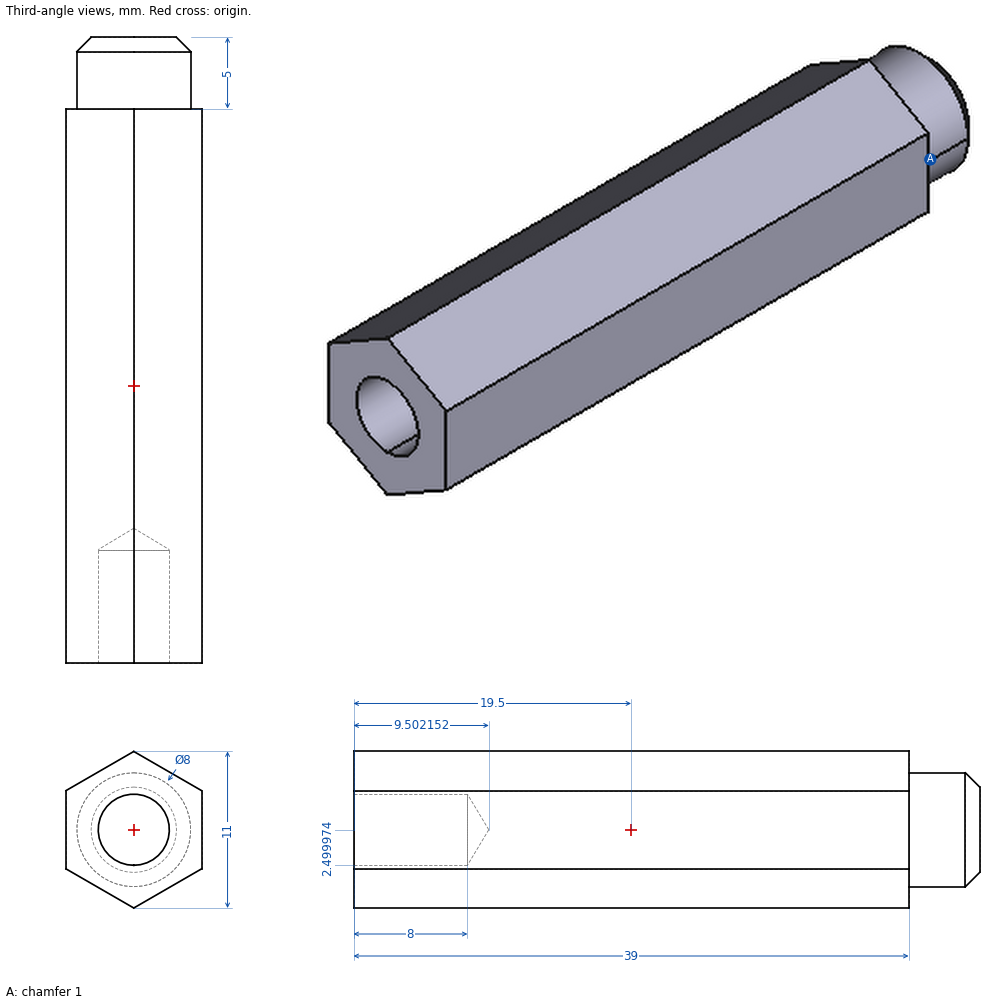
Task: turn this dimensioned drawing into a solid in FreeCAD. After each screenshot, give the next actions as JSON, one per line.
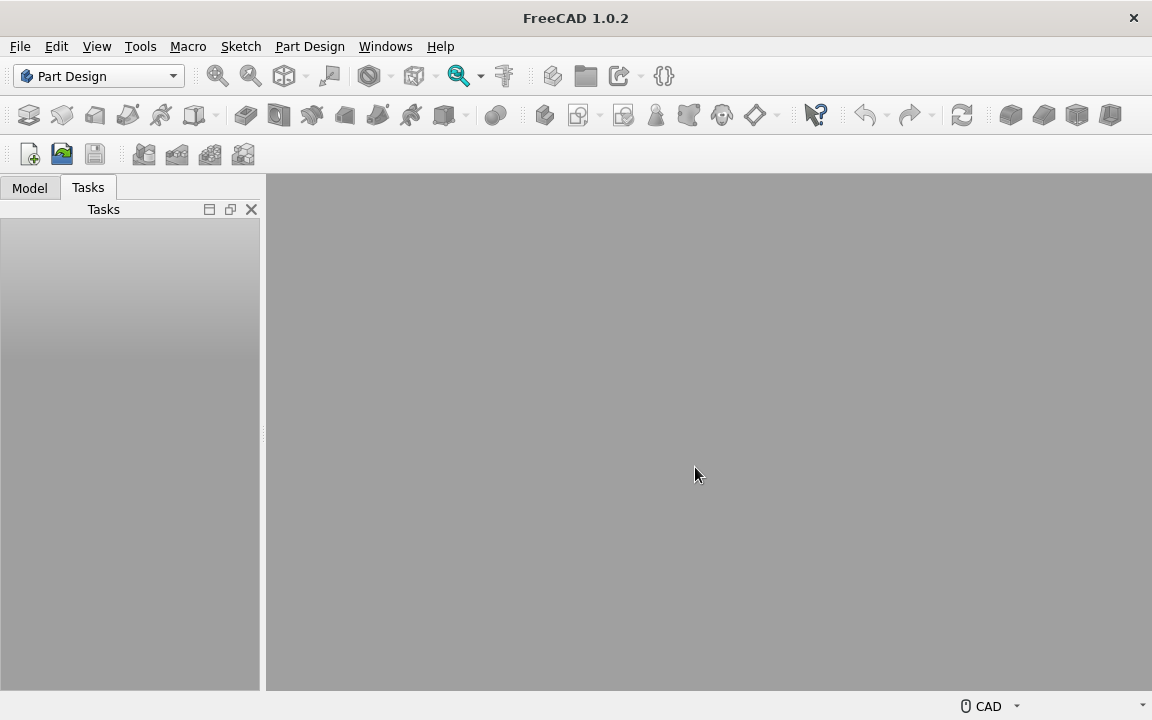
{"action": "key", "text": "ctrl+n"}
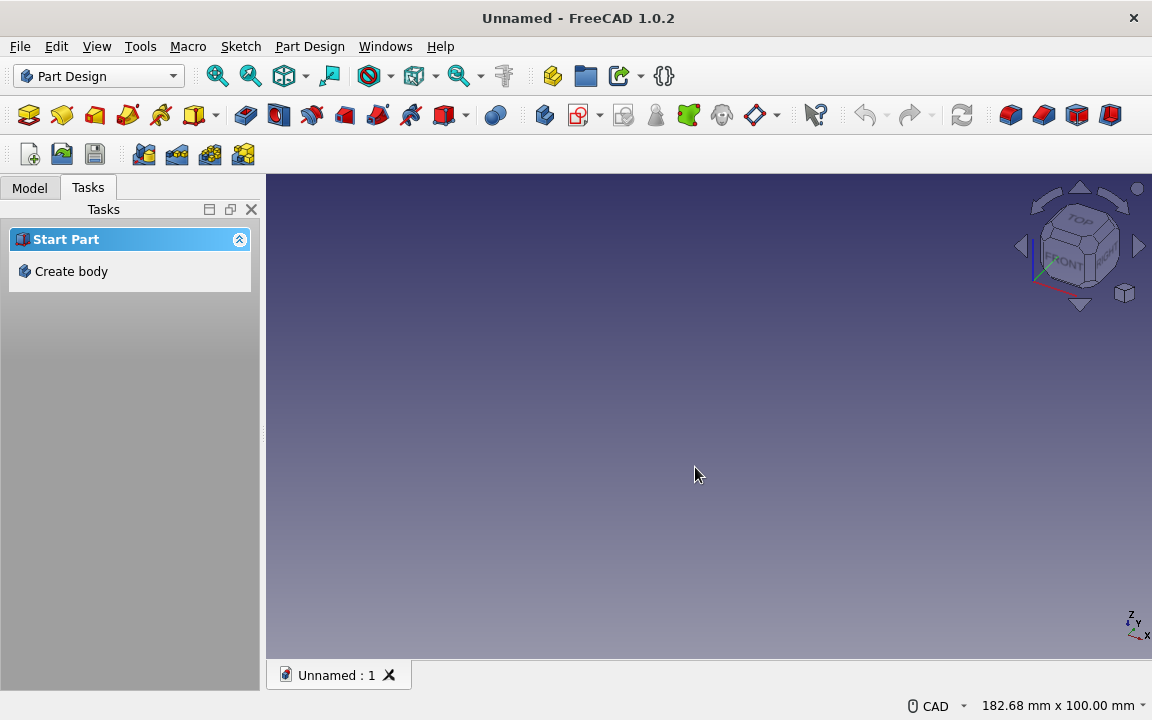
{"action": "left_click", "coordinate": [578, 116]}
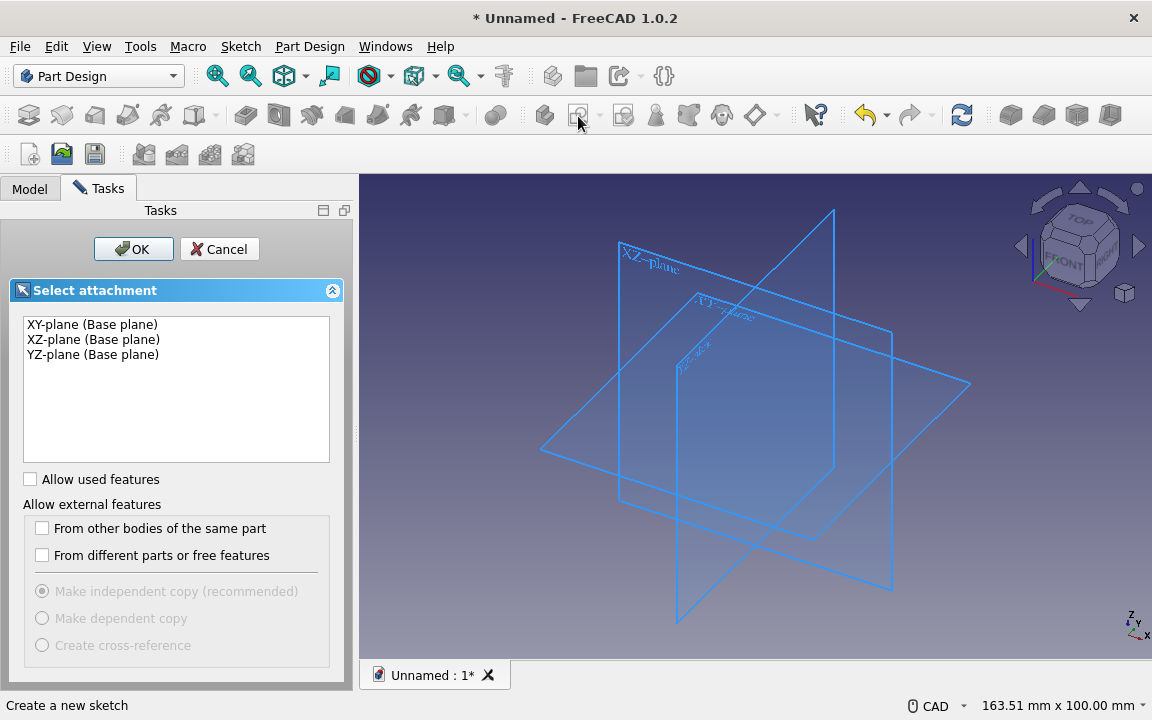
{"action": "left_click", "coordinate": [84, 340]}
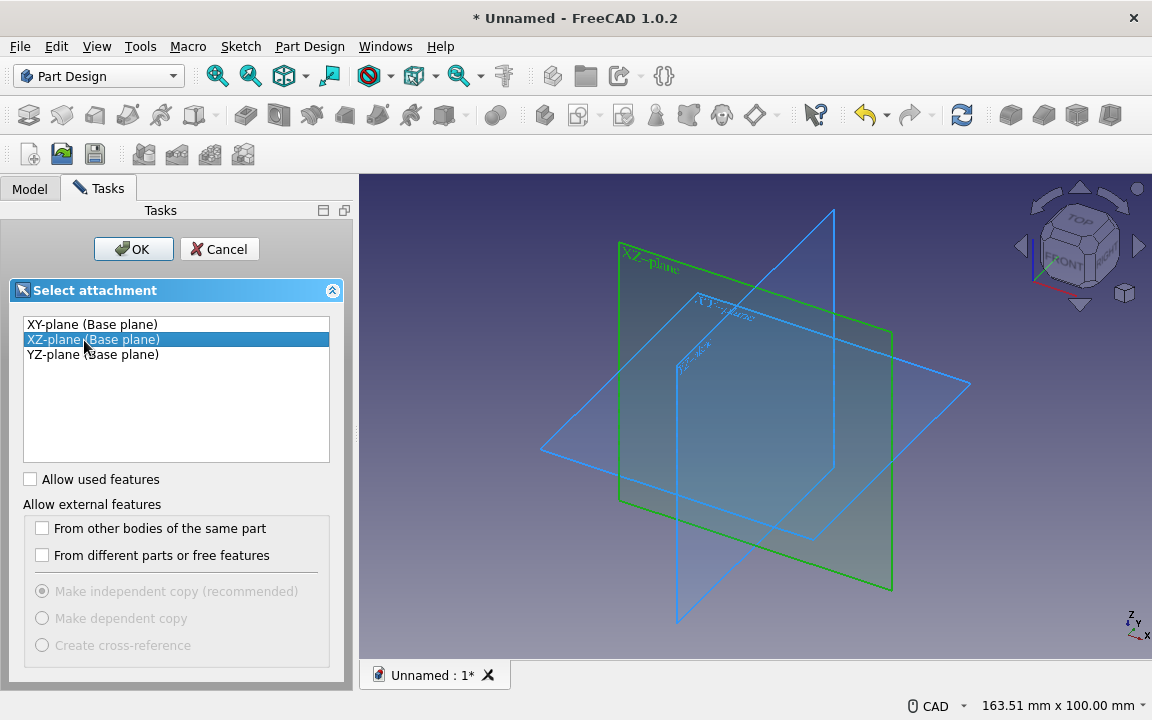
{"action": "left_click", "coordinate": [134, 249]}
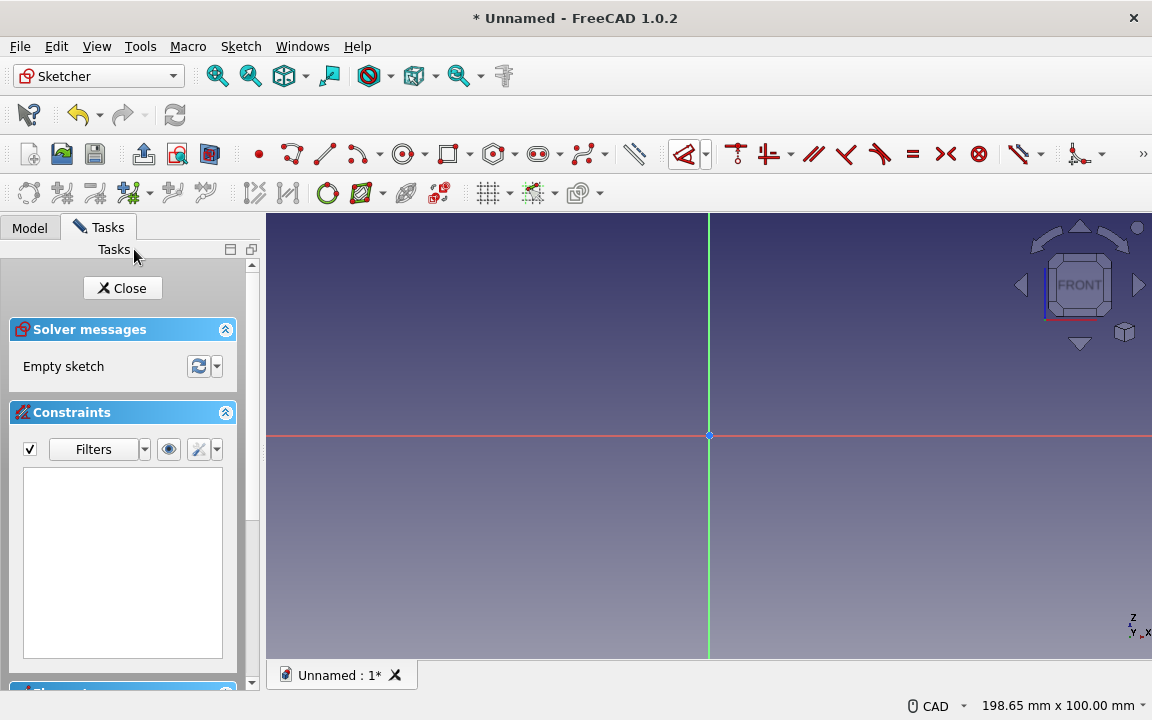
{"action": "scroll", "coordinate": [723, 436], "scroll_direction": "up", "scroll_amount": 9}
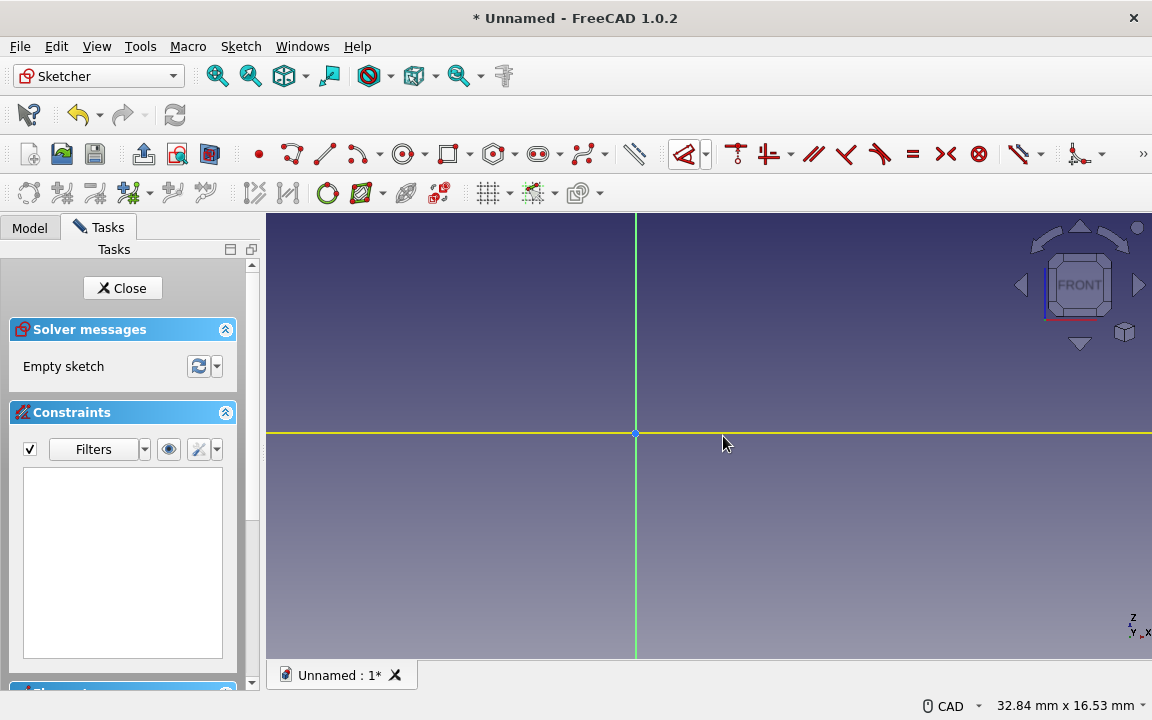
{"action": "key", "text": "g p 6"}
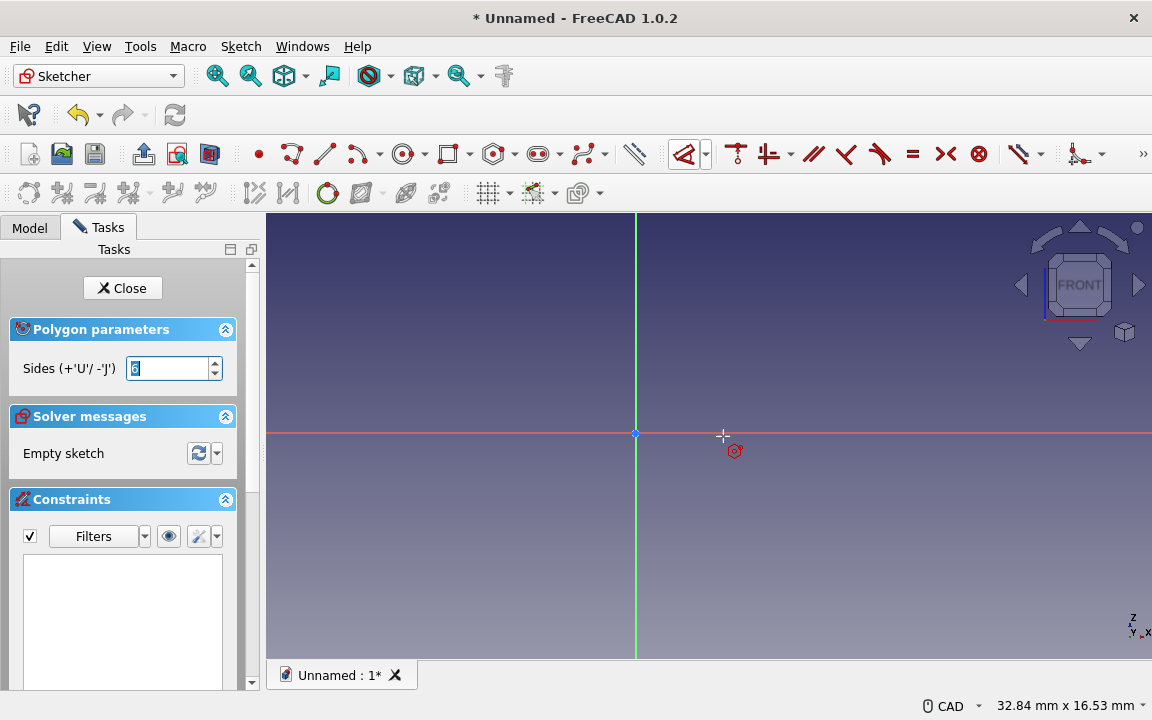
{"action": "left_click", "coordinate": [636, 433]}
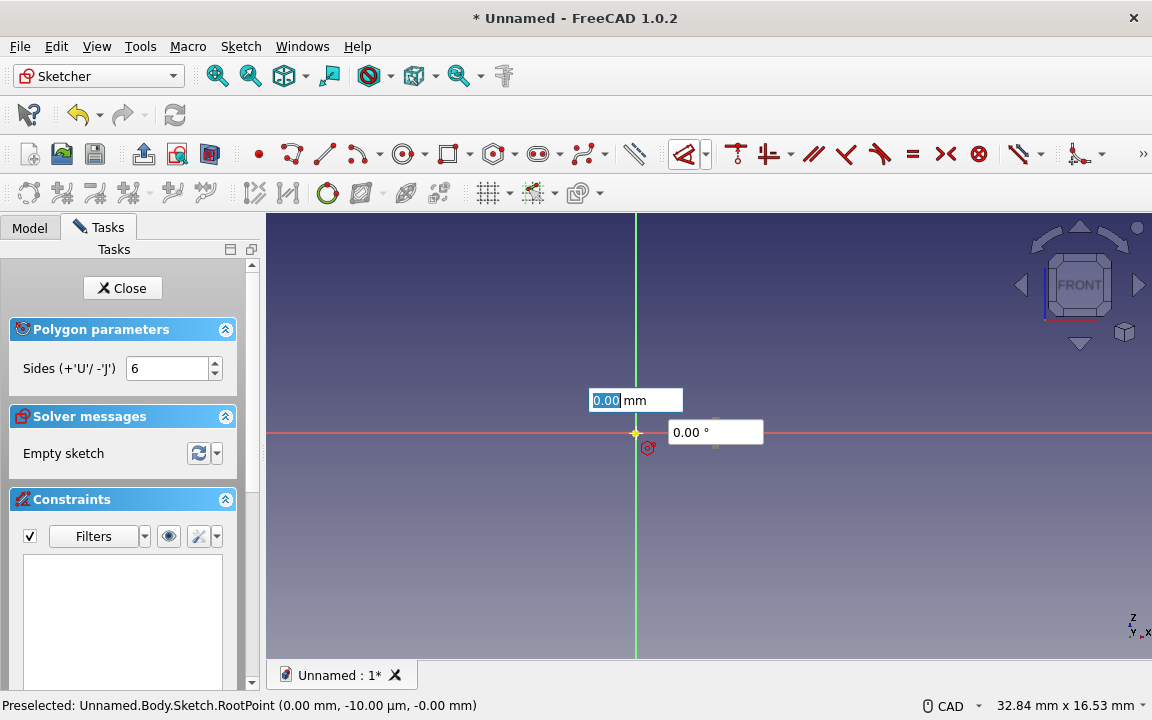
{"action": "left_click", "coordinate": [636, 582]}
{"action": "right_click", "coordinate": [636, 582]}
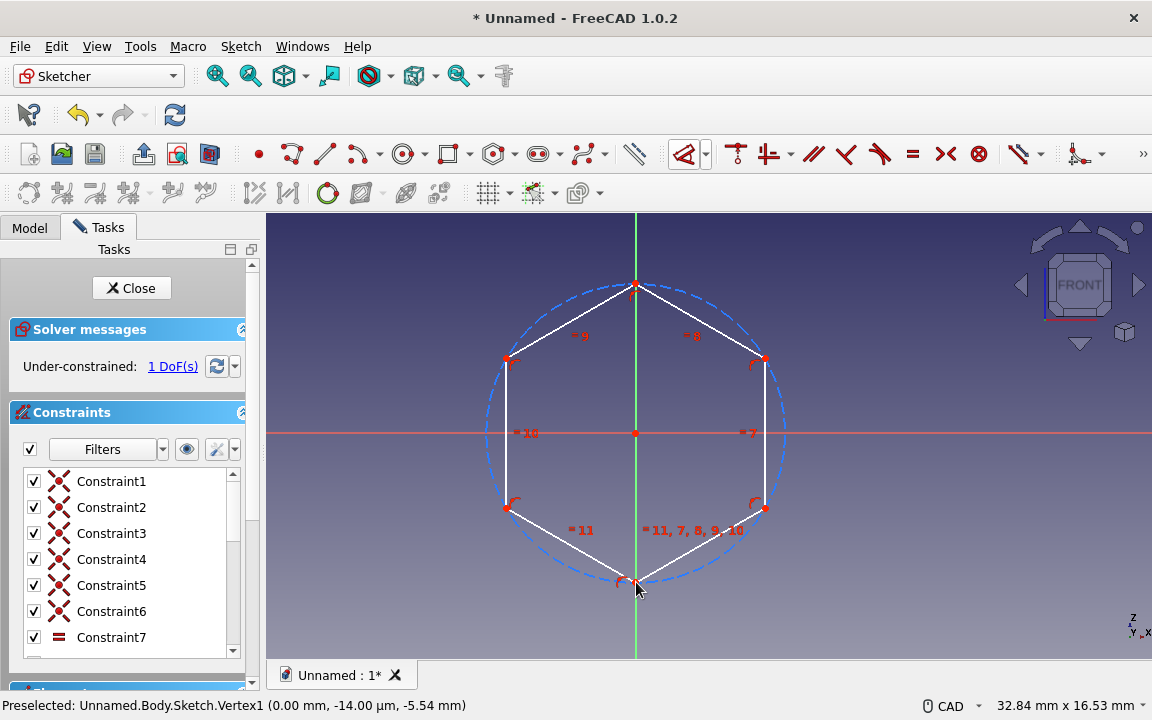
{"action": "left_click", "coordinate": [684, 154]}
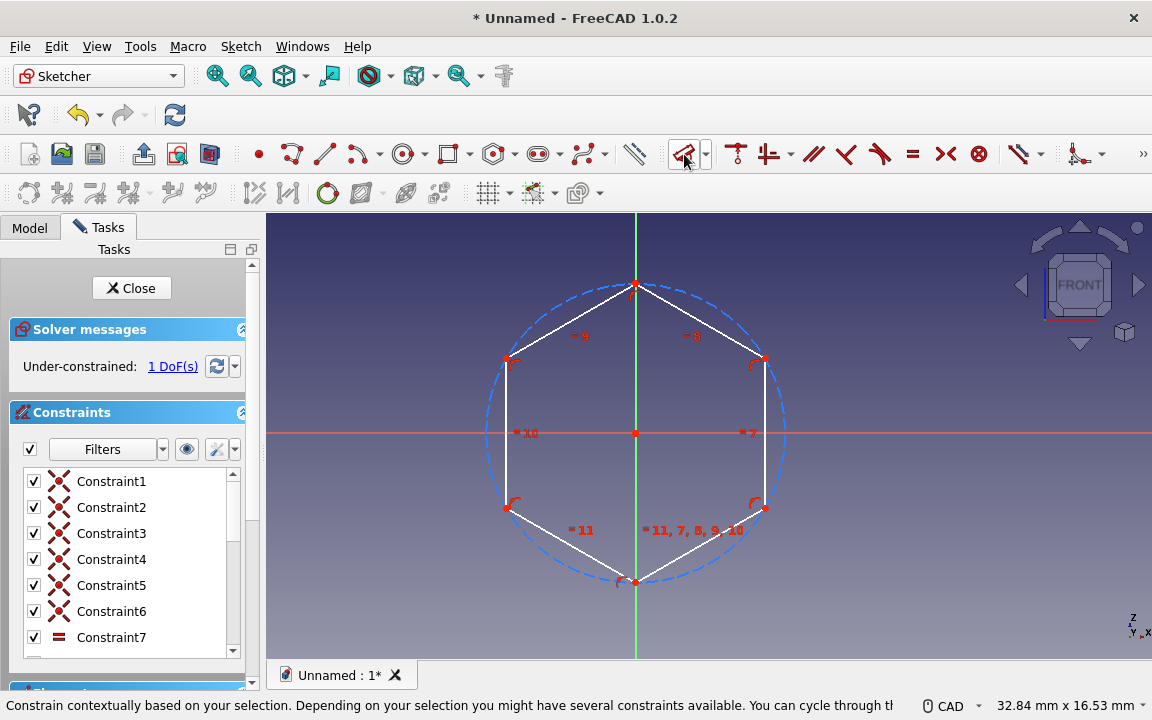
{"action": "left_click", "coordinate": [636, 583]}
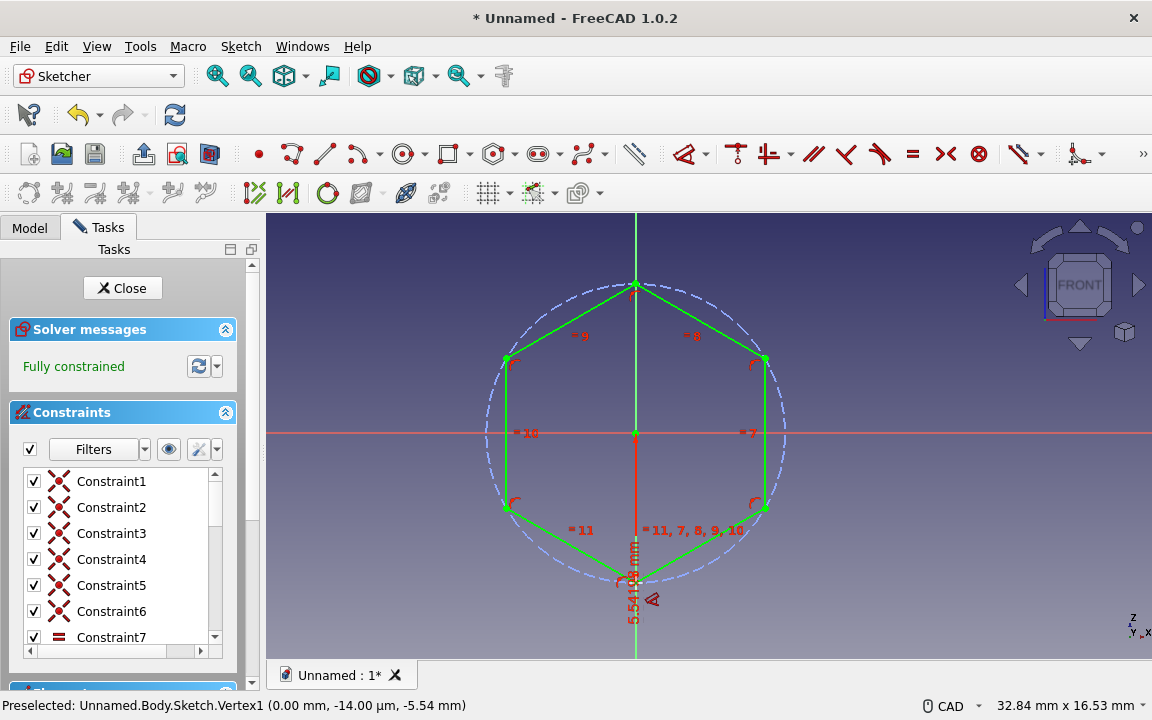
{"action": "left_click", "coordinate": [636, 284]}
{"action": "left_click", "coordinate": [670, 365]}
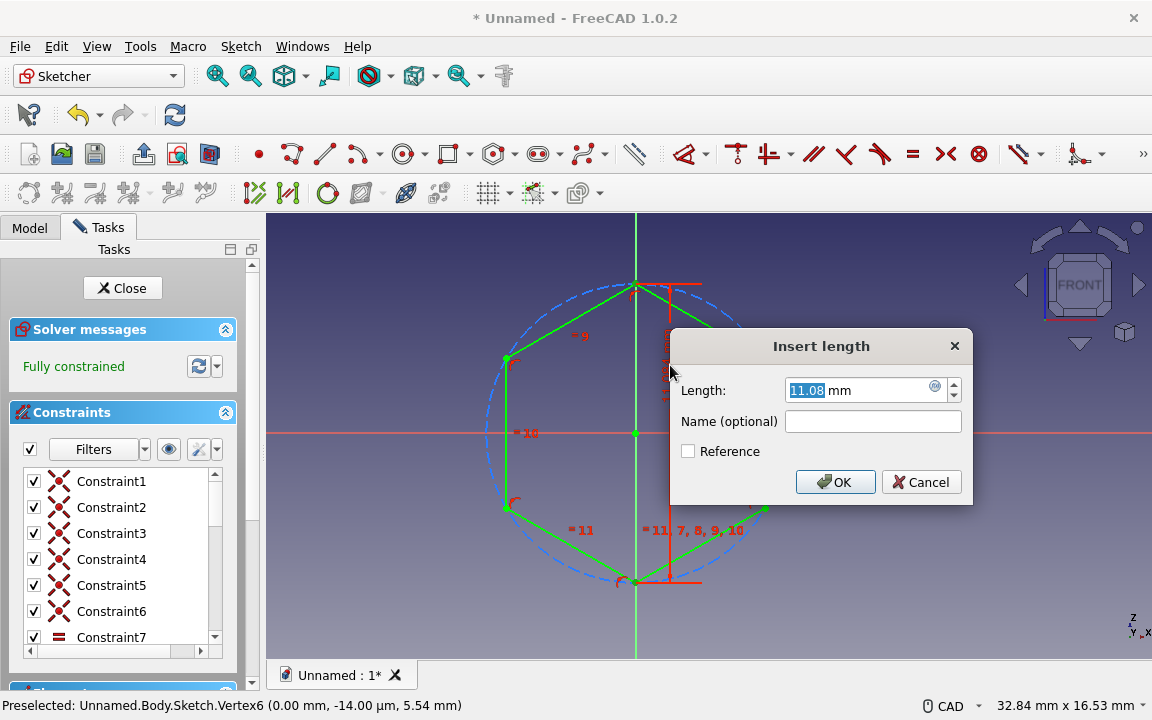
{"action": "type", "text": "11"}
{"action": "key", "text": "Return"}
{"action": "key", "text": "Escape"}